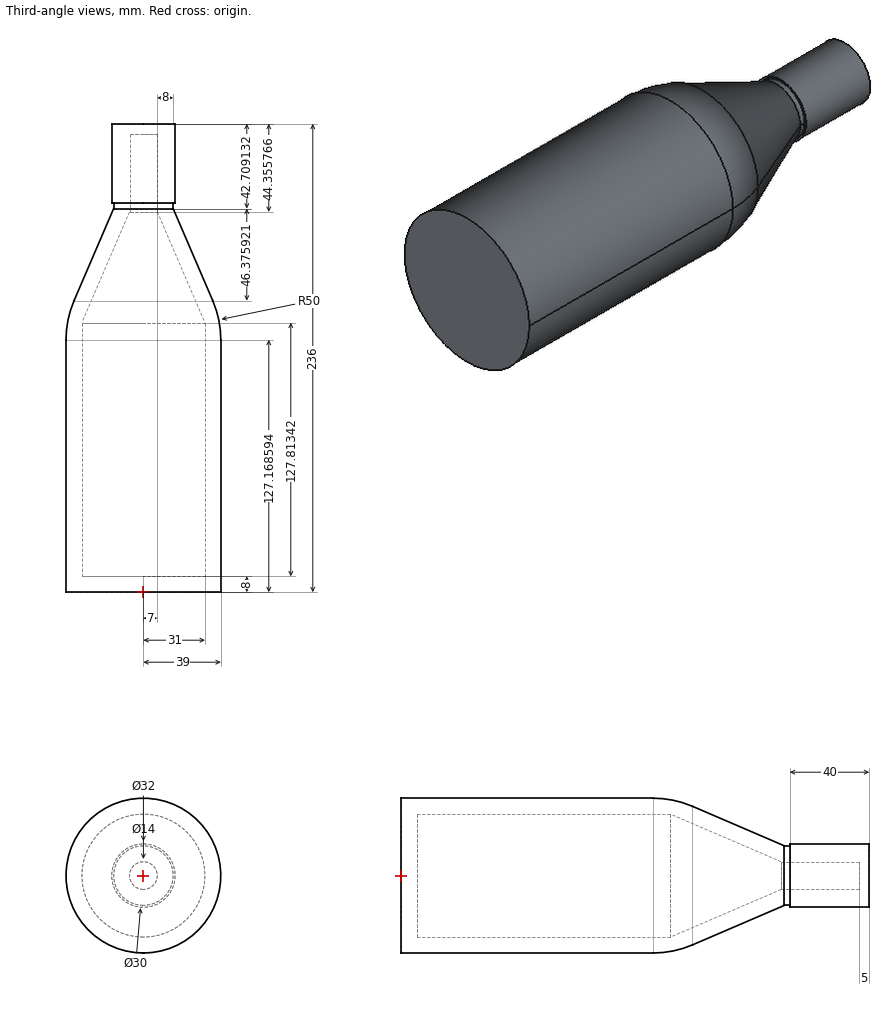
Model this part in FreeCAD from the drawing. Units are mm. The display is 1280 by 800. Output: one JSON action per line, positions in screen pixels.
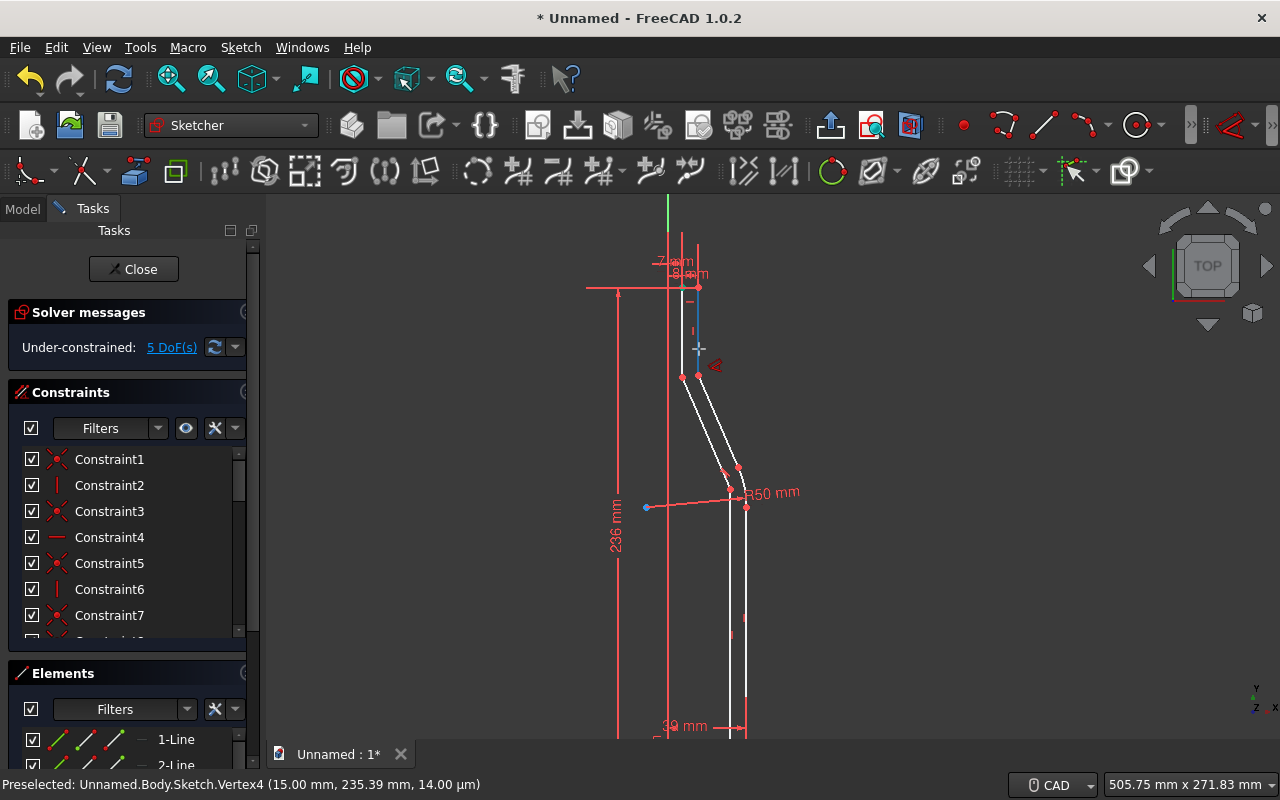
{"action": "left_click", "coordinate": [698, 349]}
{"action": "left_click", "coordinate": [732, 332]}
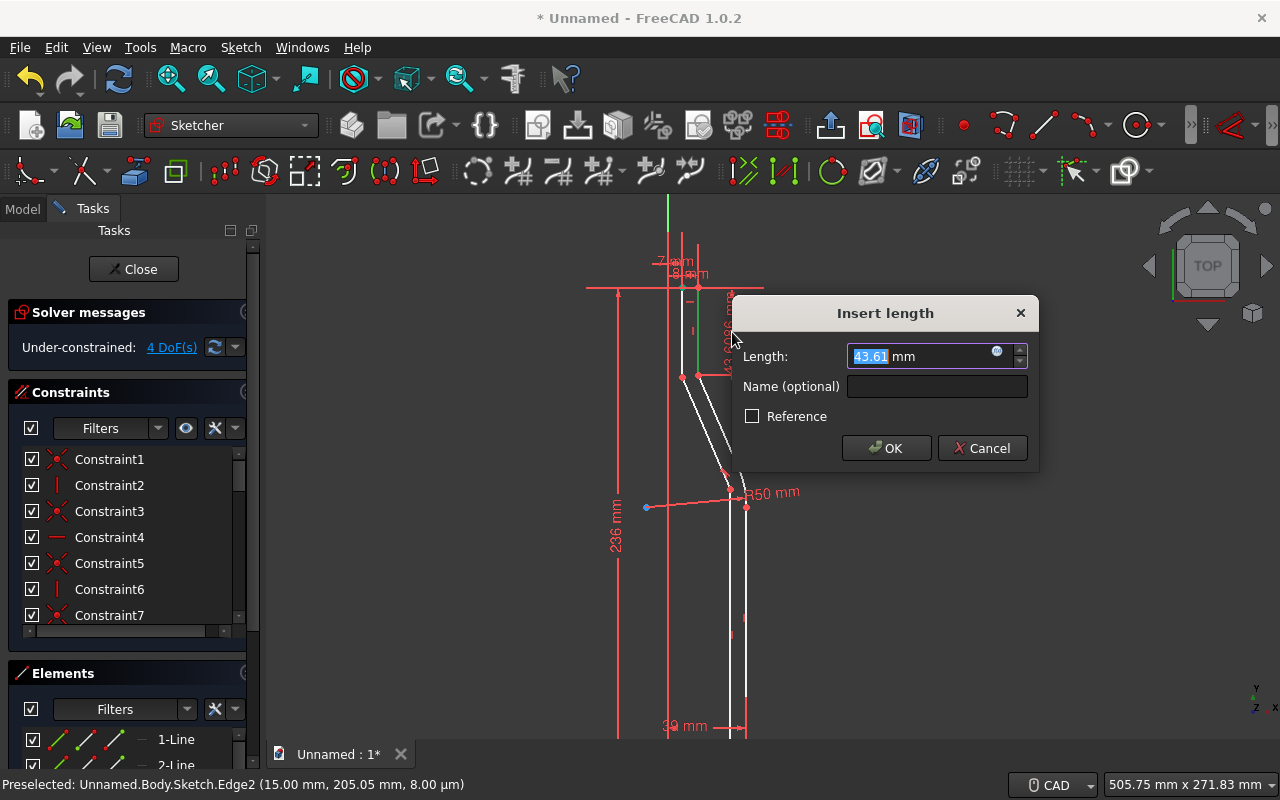
{"action": "type", "text": "42.709132"}
{"action": "key", "text": "Return"}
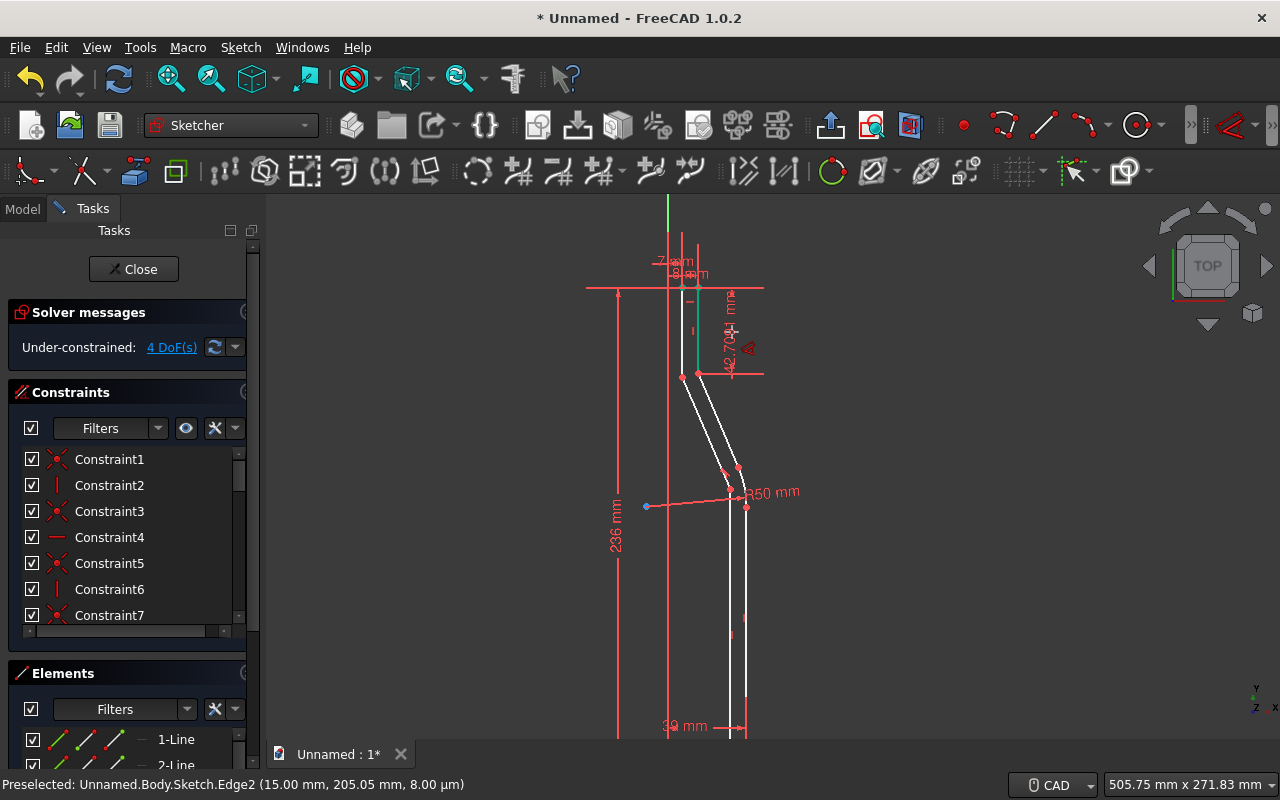
{"action": "left_click", "coordinate": [682, 315]}
{"action": "left_click", "coordinate": [648, 333]}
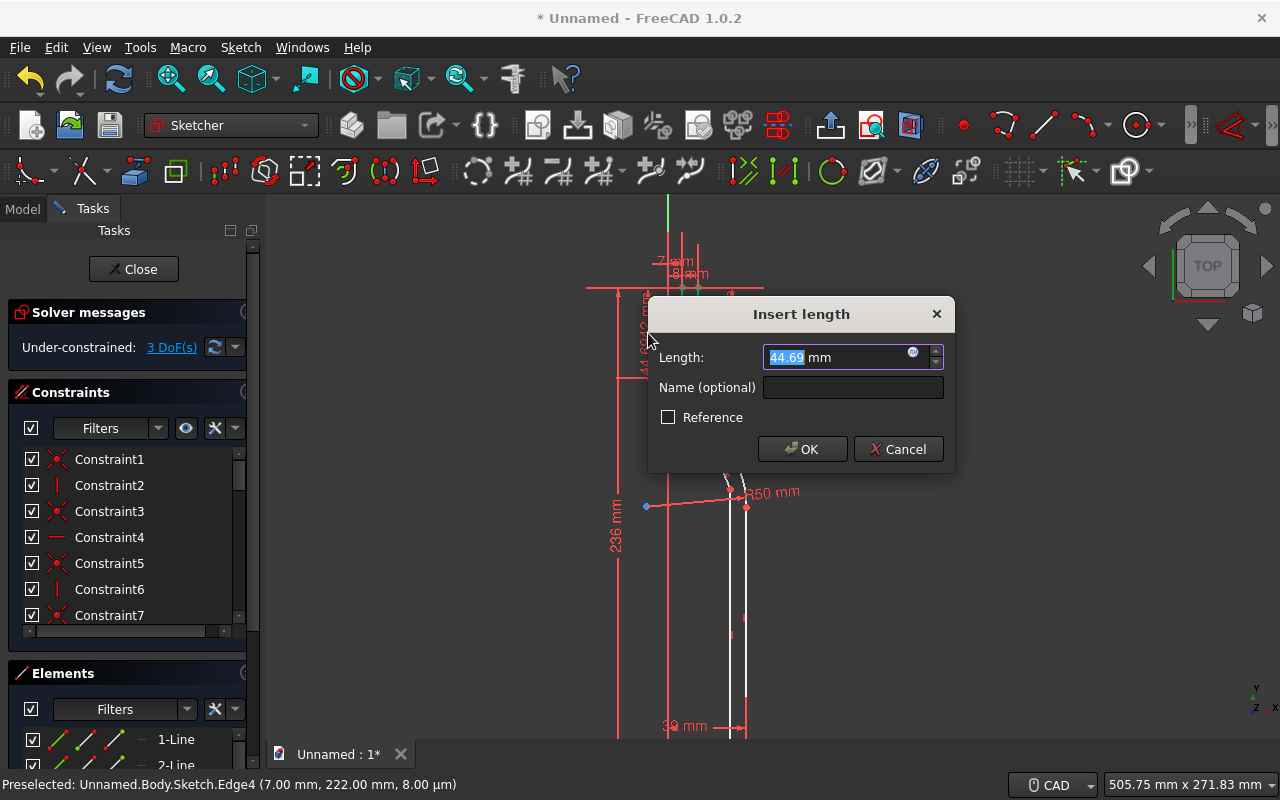
{"action": "type", "text": "44.355766"}
{"action": "key", "text": "Return"}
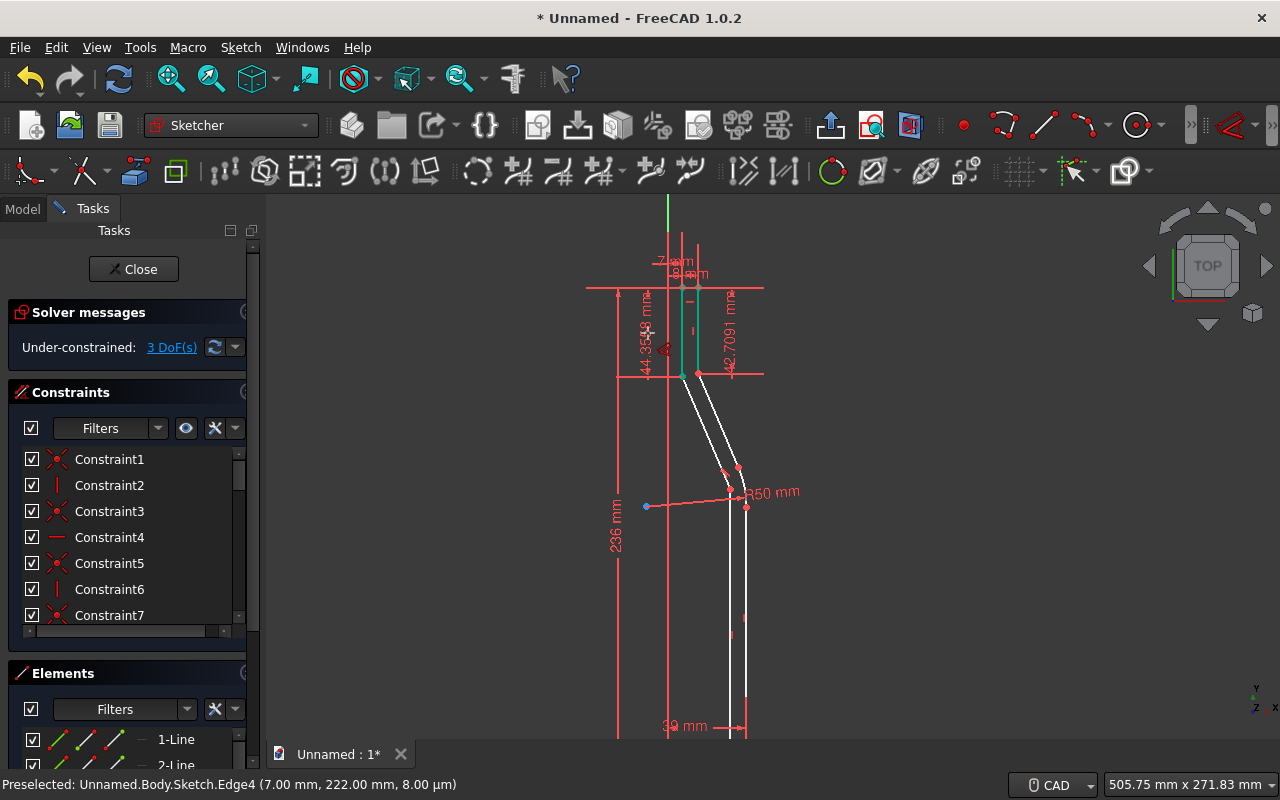
{"action": "left_click", "coordinate": [730, 566]}
{"action": "left_click", "coordinate": [764, 600]}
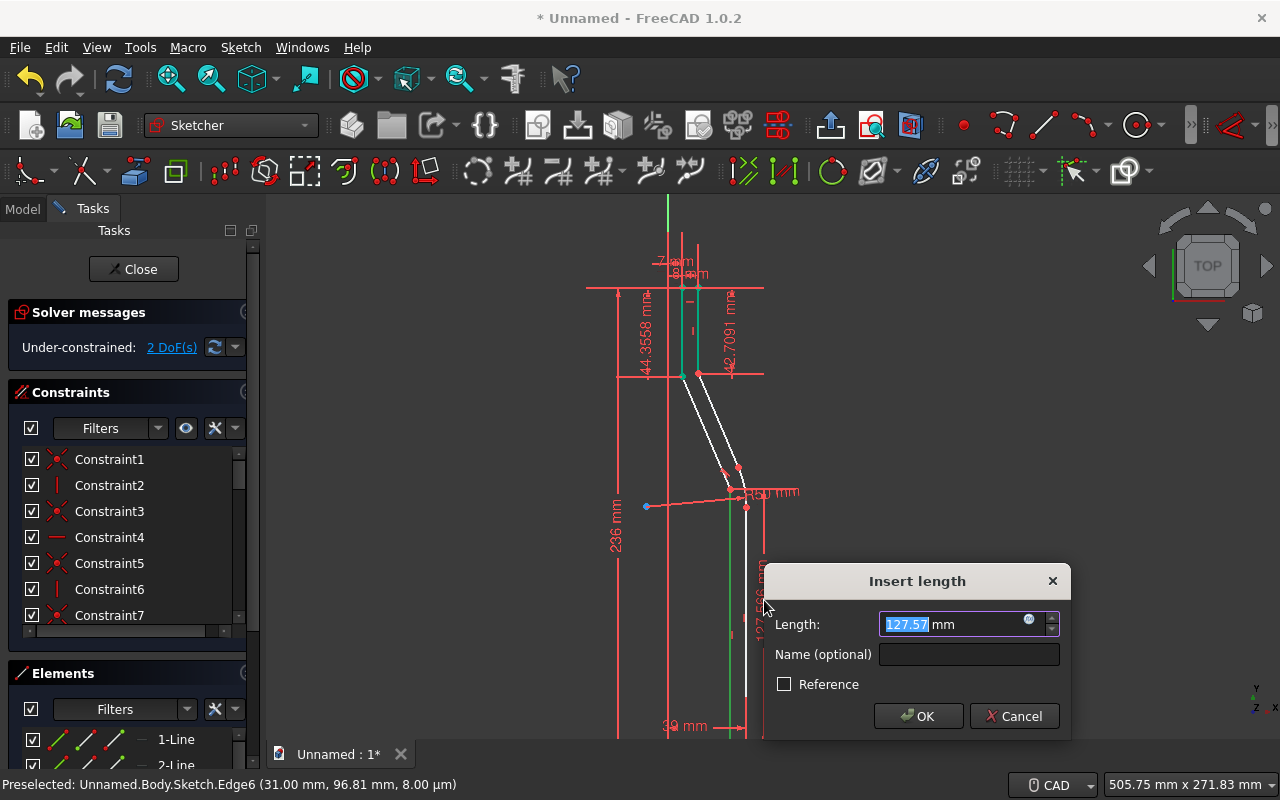
{"action": "type", "text": "127.81342"}
{"action": "key", "text": "Return"}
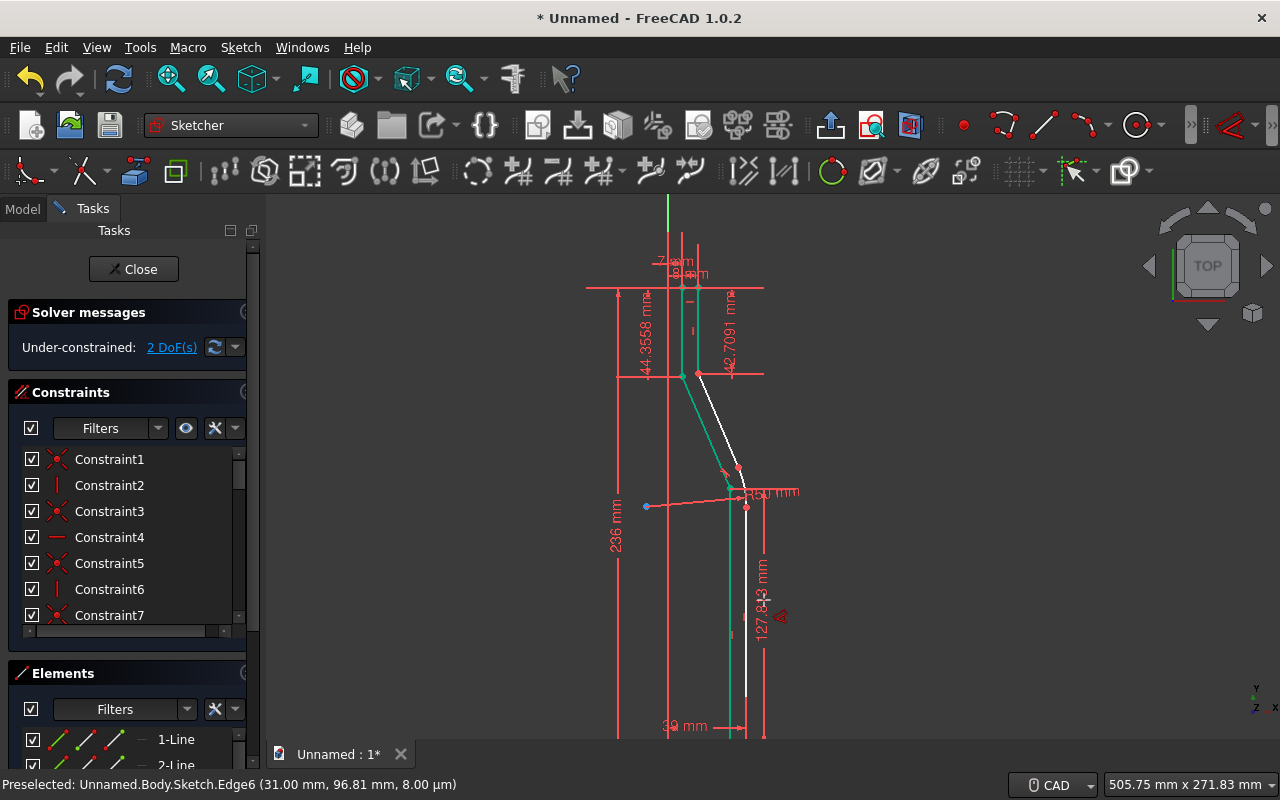
{"action": "left_click", "coordinate": [746, 685]}
{"action": "left_click", "coordinate": [780, 563]}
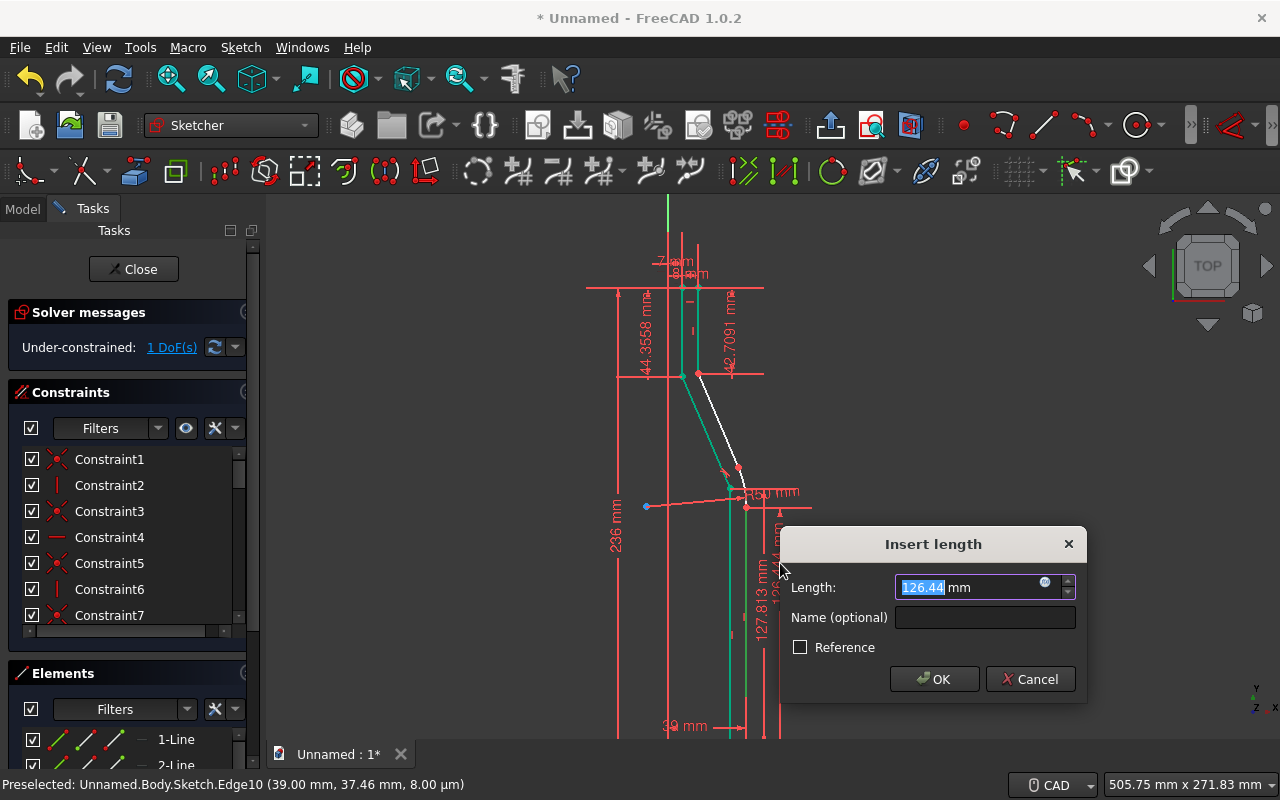
{"action": "type", "text": "127.168594"}
{"action": "key", "text": "Return"}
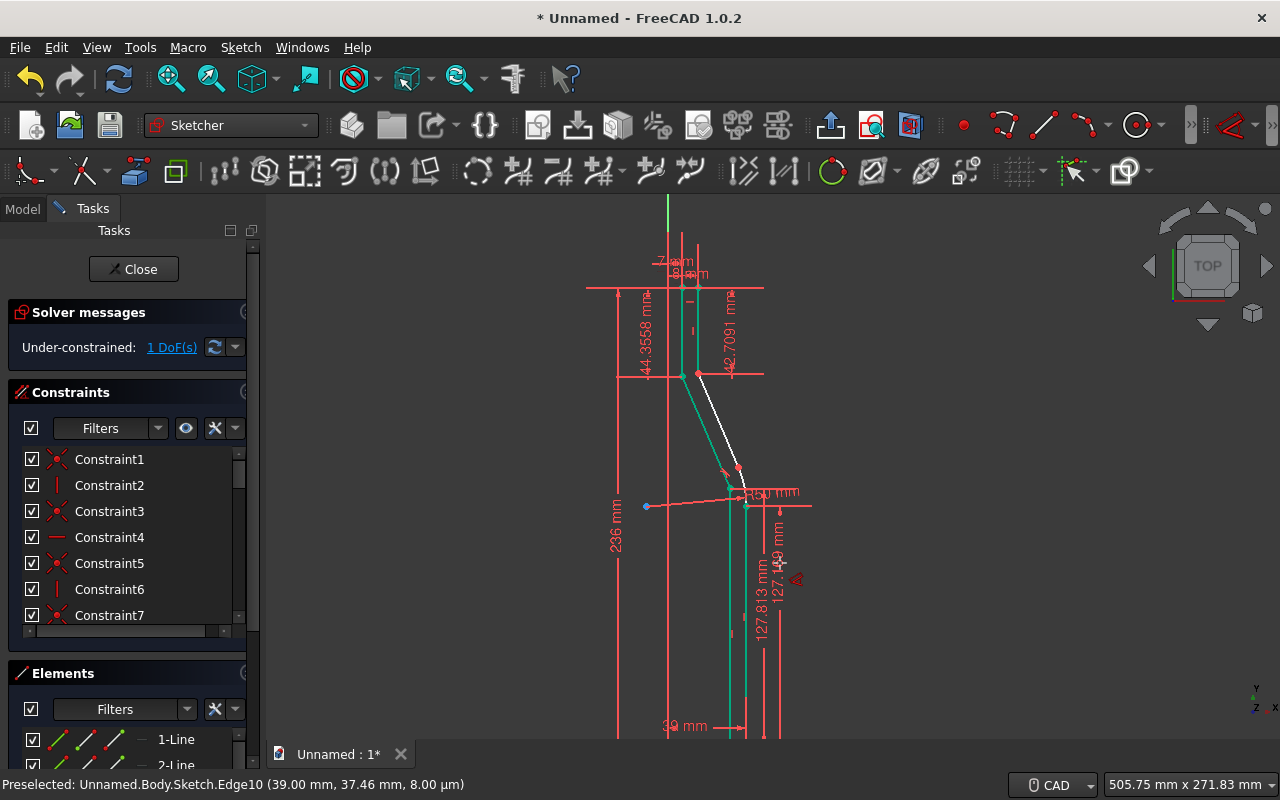
{"action": "left_click", "coordinate": [726, 439]}
{"action": "left_click", "coordinate": [772, 421]}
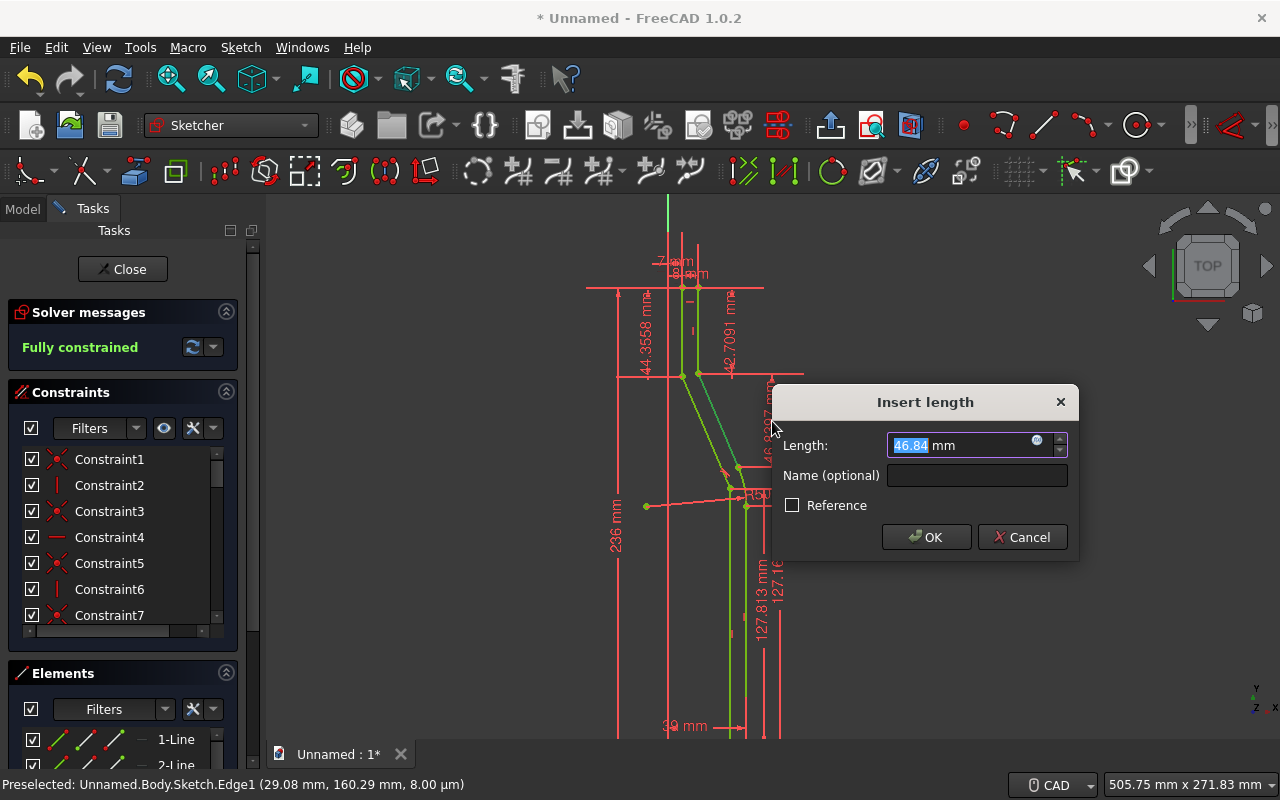
{"action": "type", "text": "46.375921"}
{"action": "key", "text": "Return"}
{"action": "key", "text": "Escape"}